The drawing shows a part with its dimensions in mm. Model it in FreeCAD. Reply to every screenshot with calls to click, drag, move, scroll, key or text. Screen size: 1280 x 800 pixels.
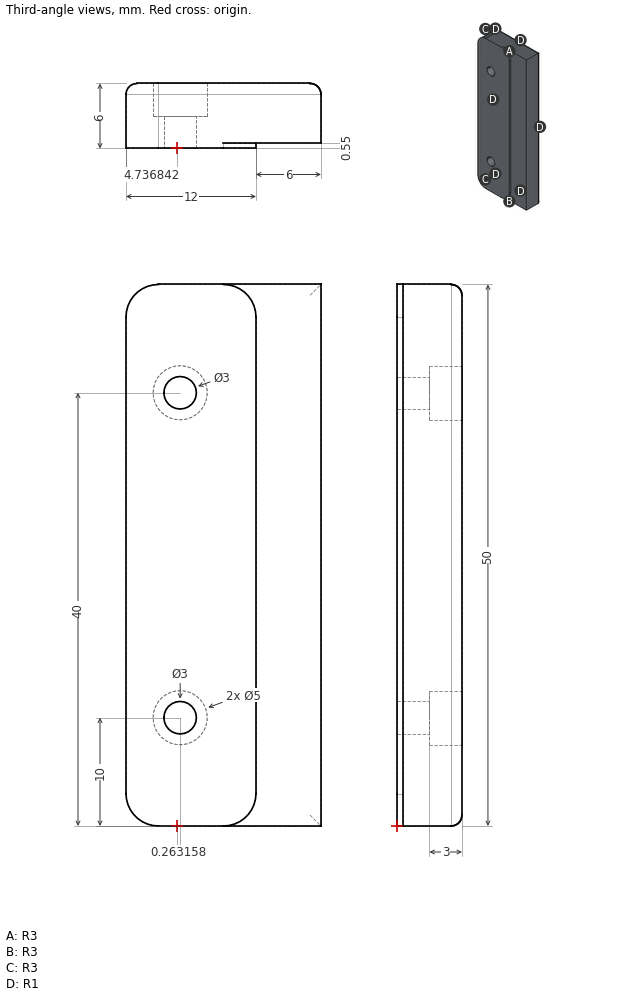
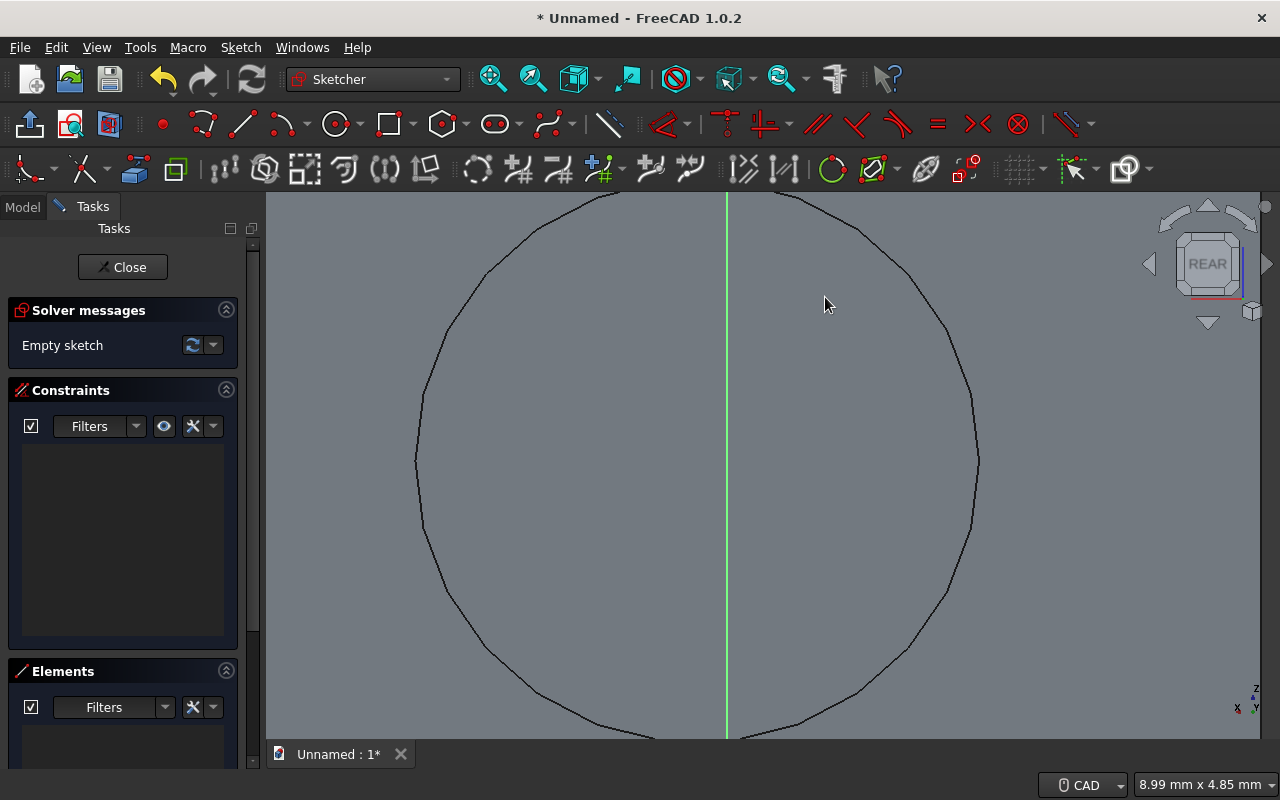
click(336, 124)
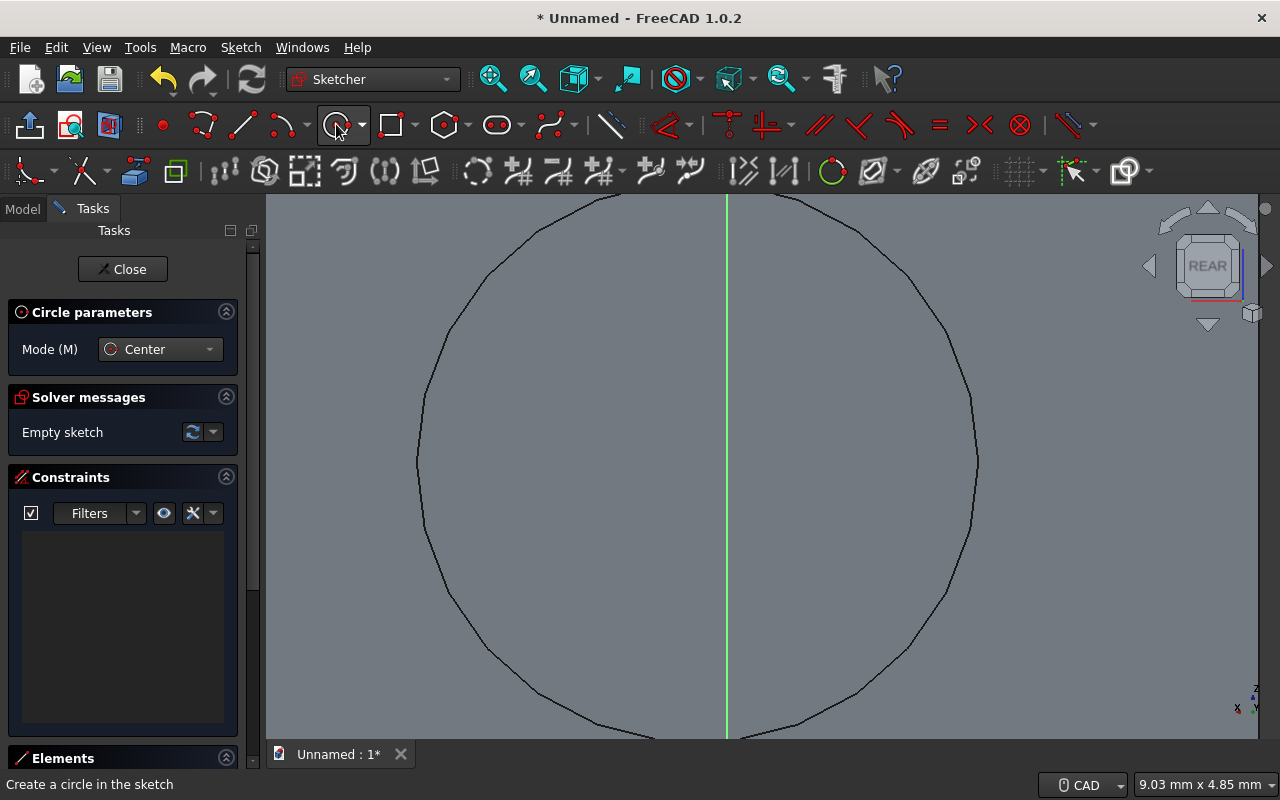
click(698, 462)
click(817, 343)
key(Escape)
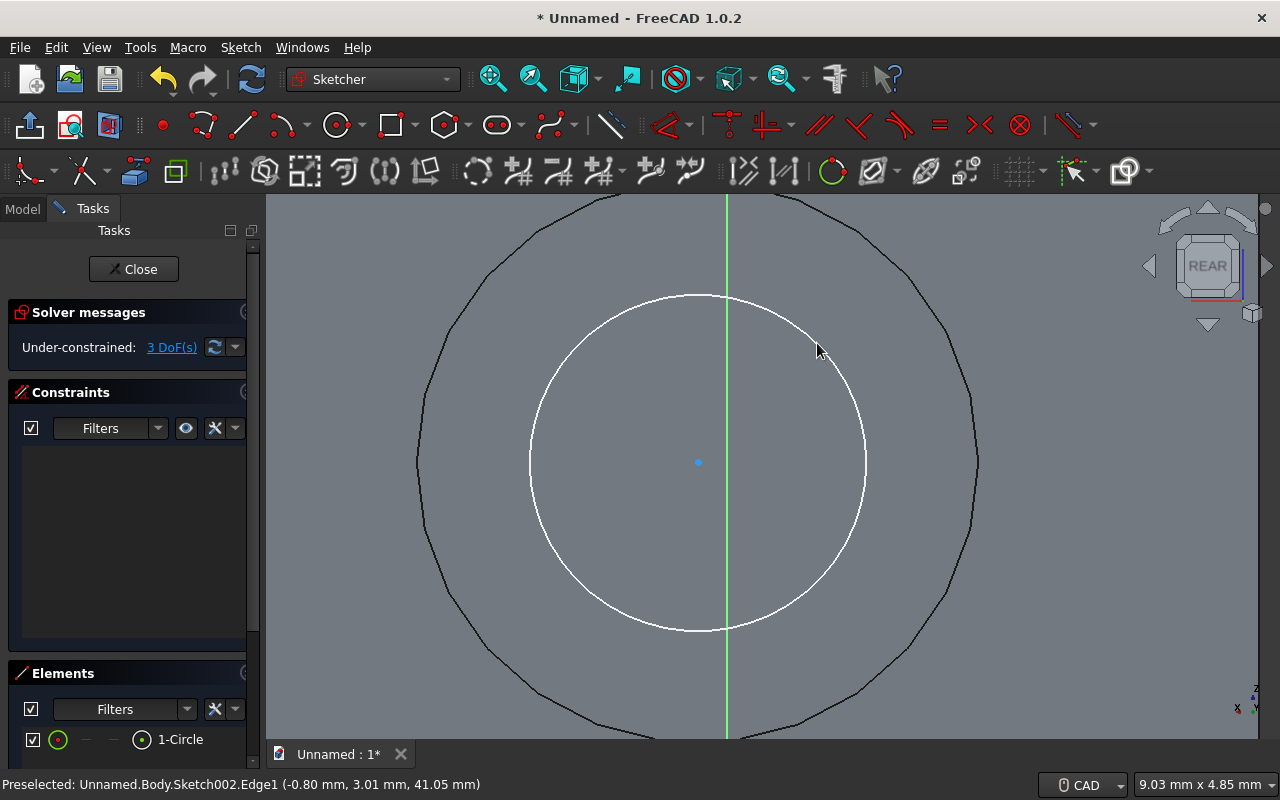
click(666, 126)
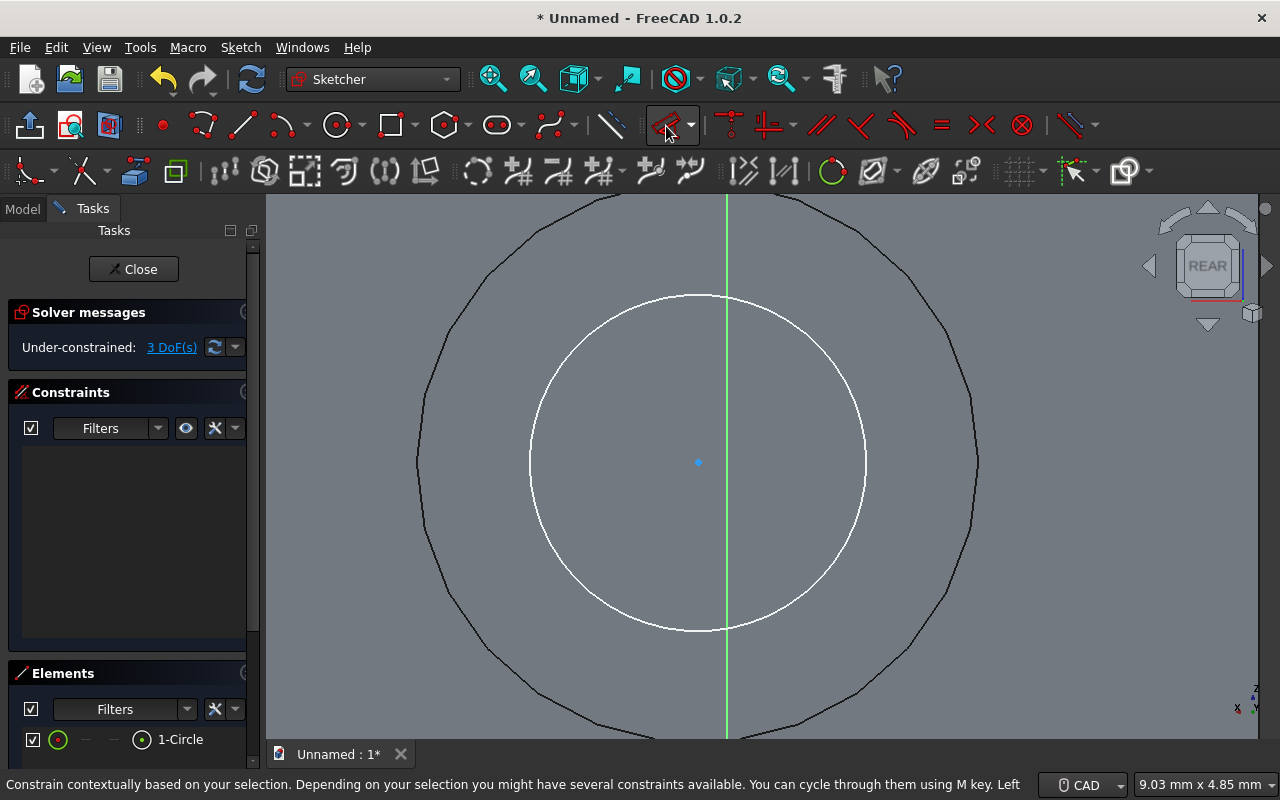
click(817, 344)
click(840, 321)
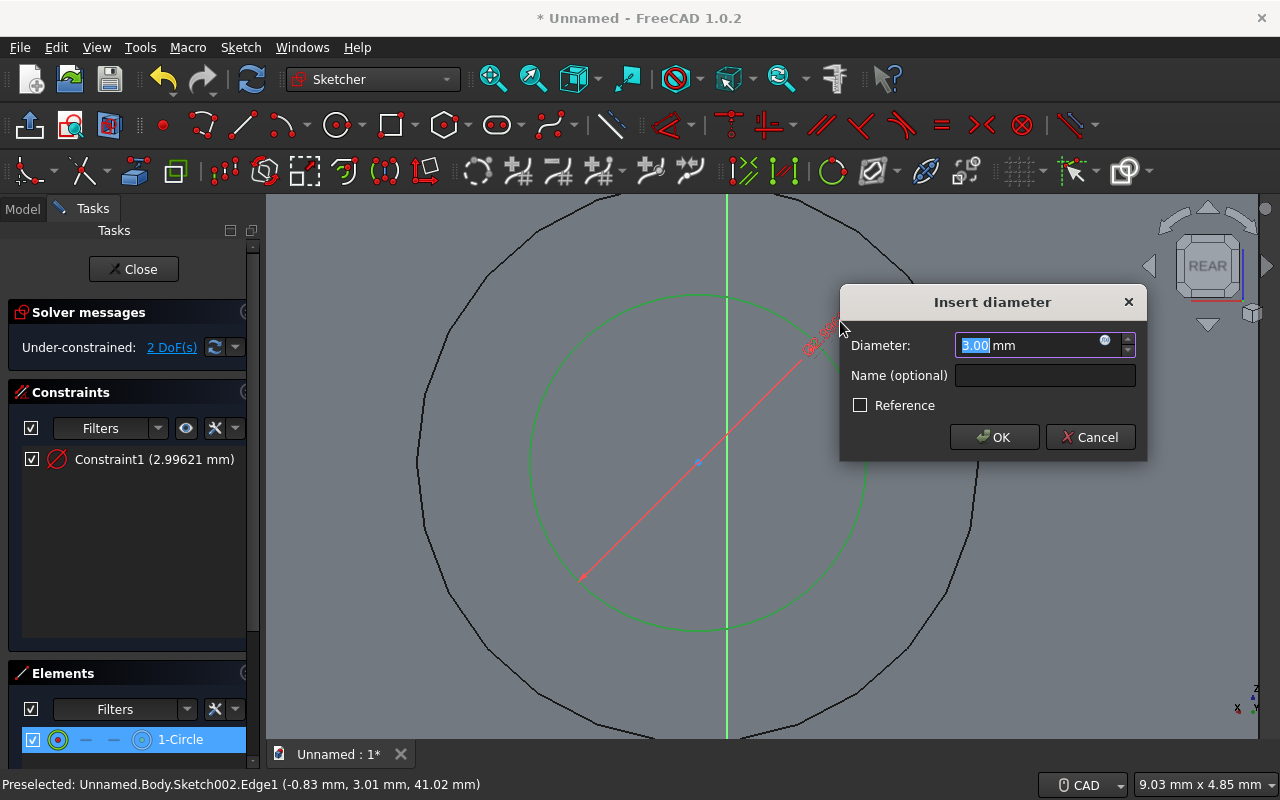
text(3)
key(Return)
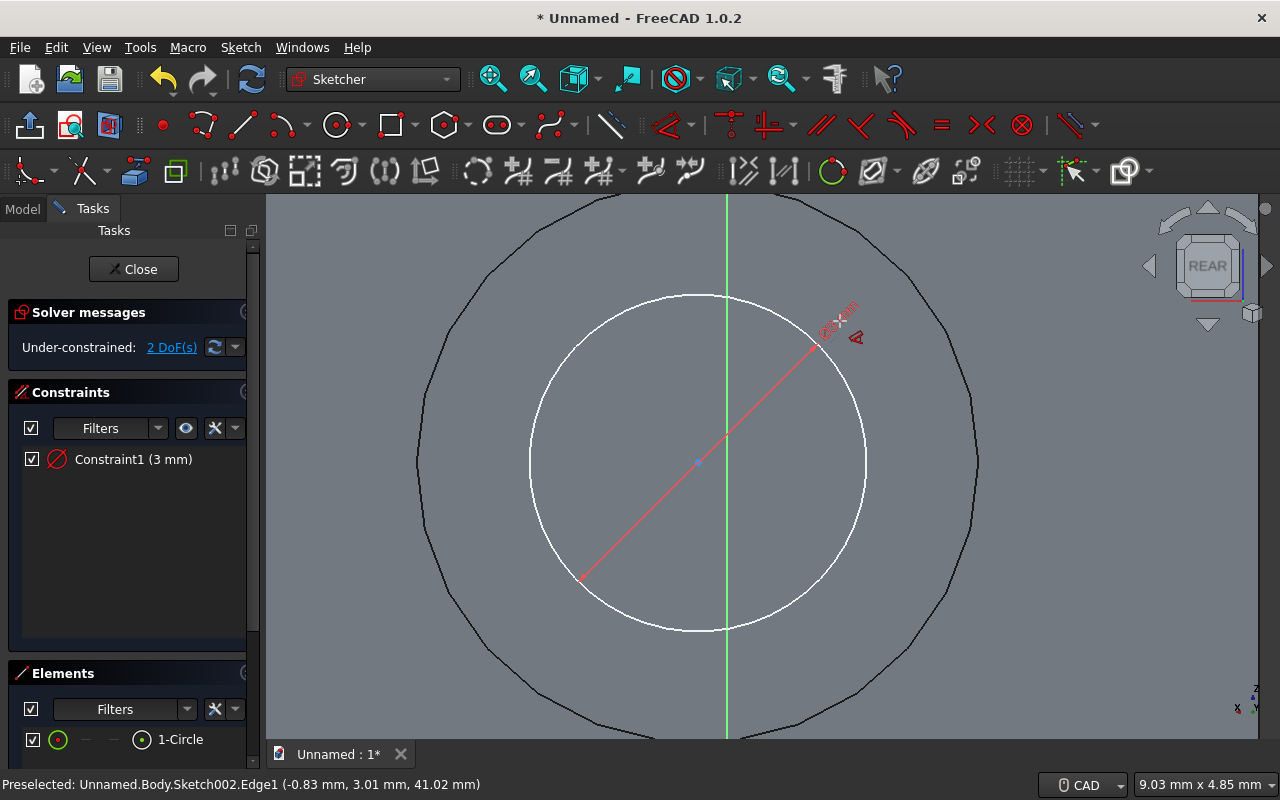
click(698, 463)
click(761, 587)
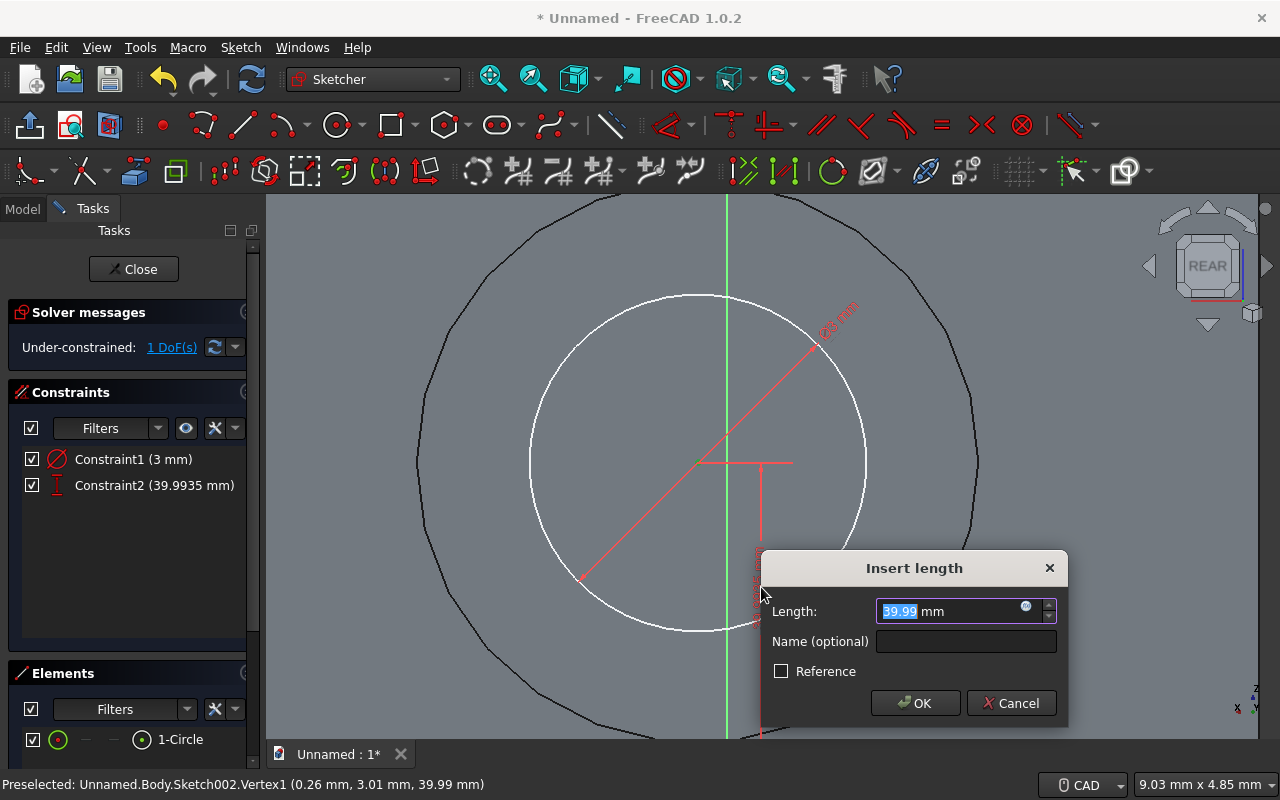
text(40)
key(Return)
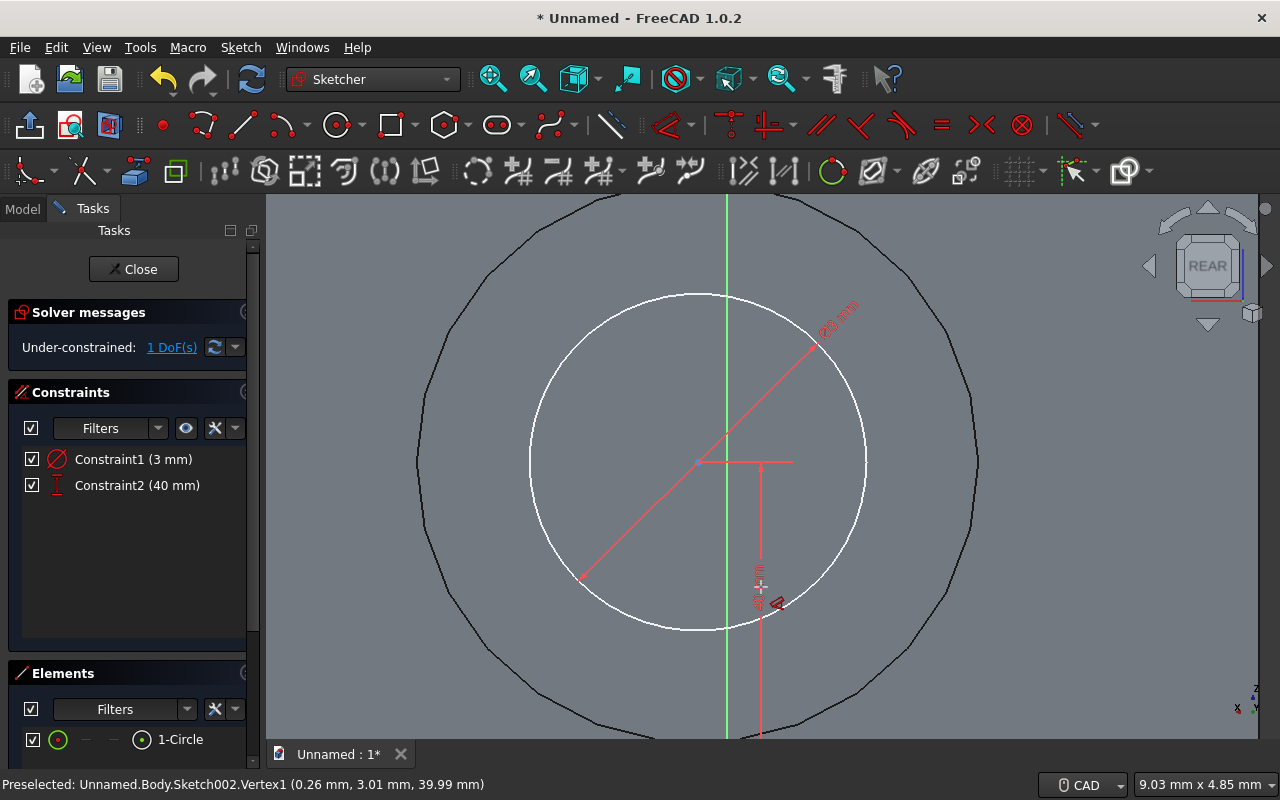
scroll(698, 462, up, 2)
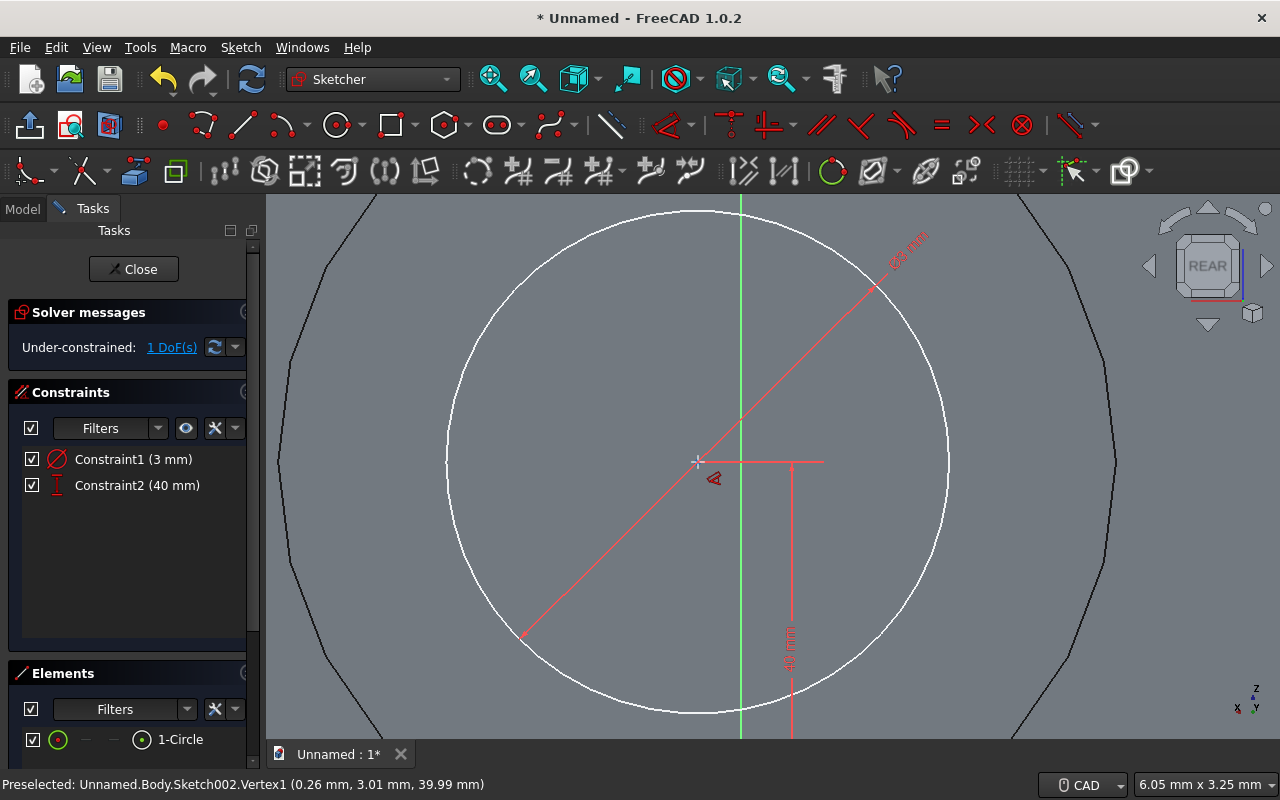
click(698, 462)
click(719, 428)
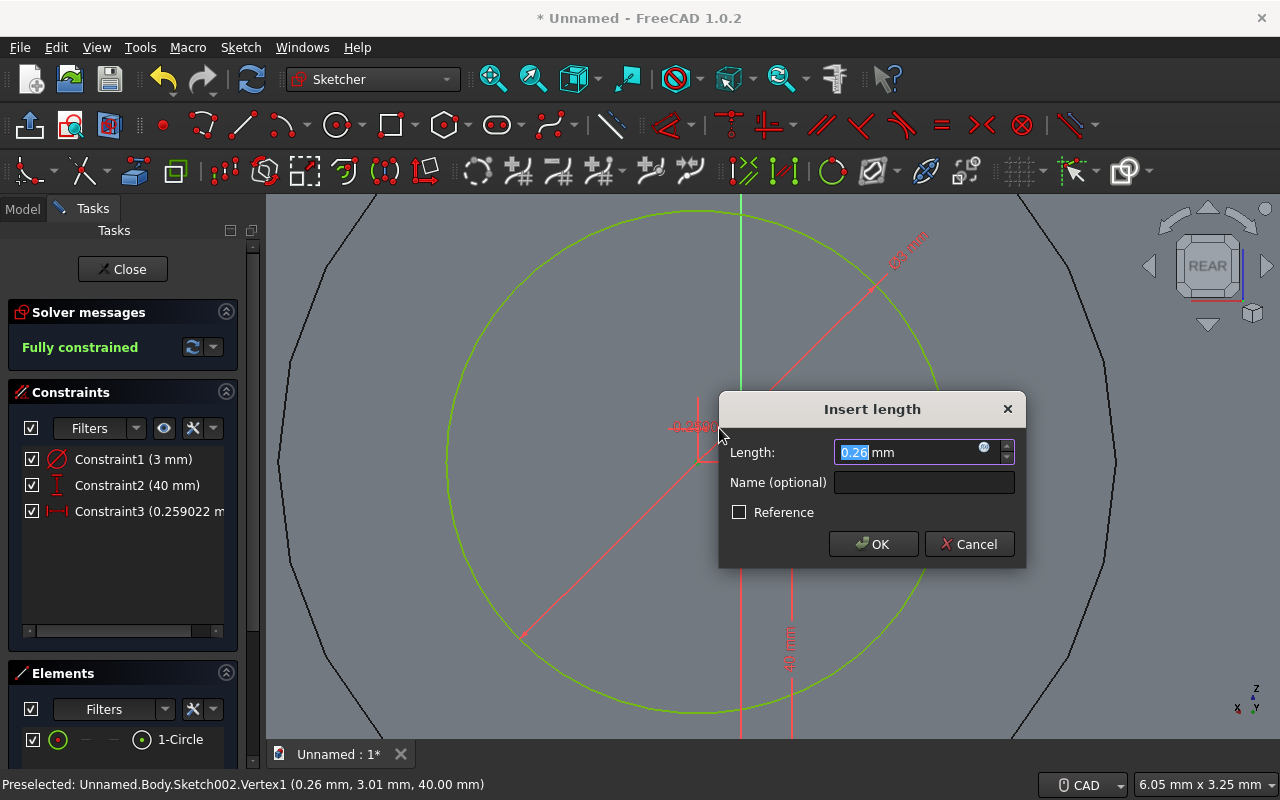
text(0.263158)
key(Return)
key(Escape)